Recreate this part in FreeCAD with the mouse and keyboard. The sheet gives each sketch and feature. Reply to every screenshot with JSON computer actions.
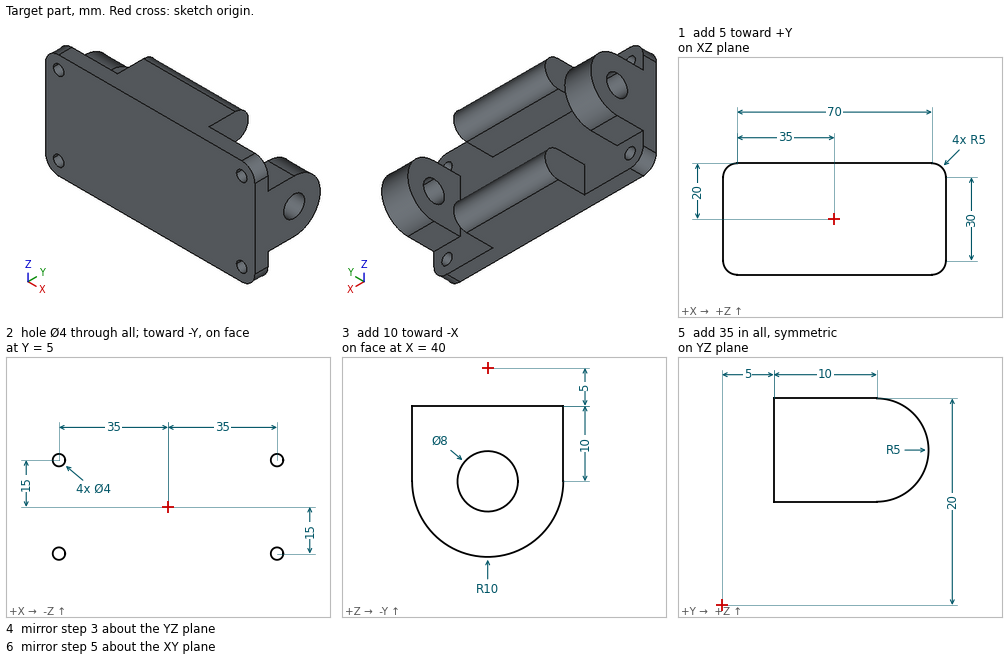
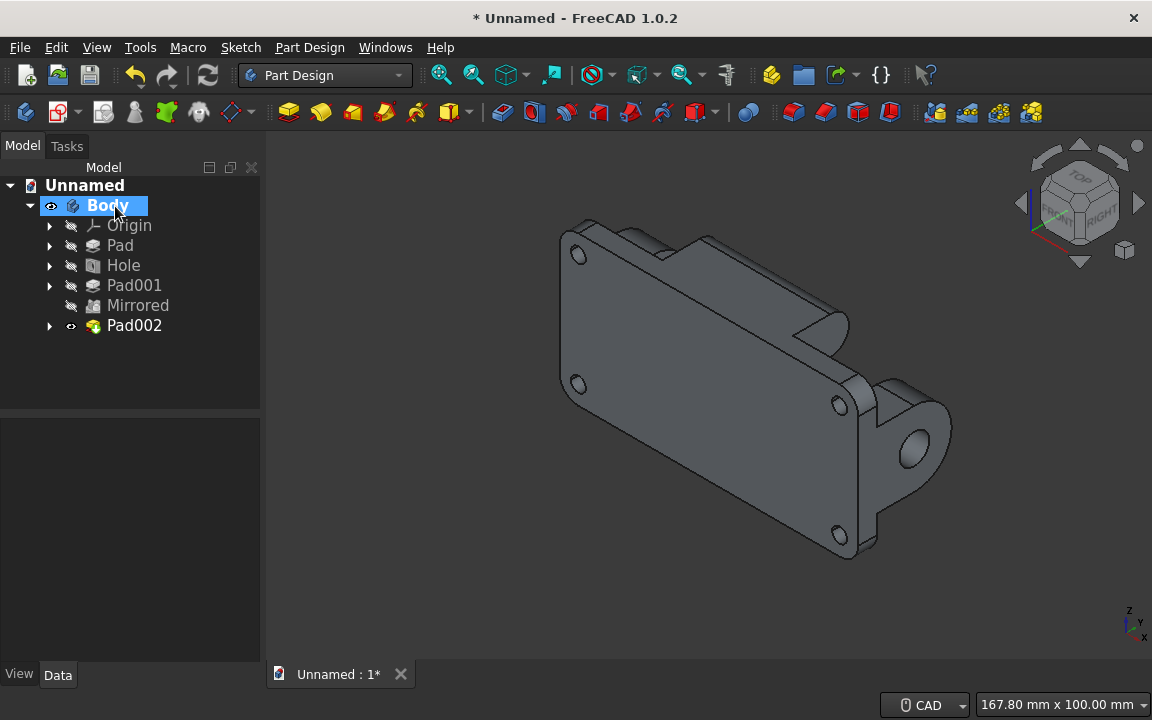
{"action": "left_click", "coordinate": [116, 326]}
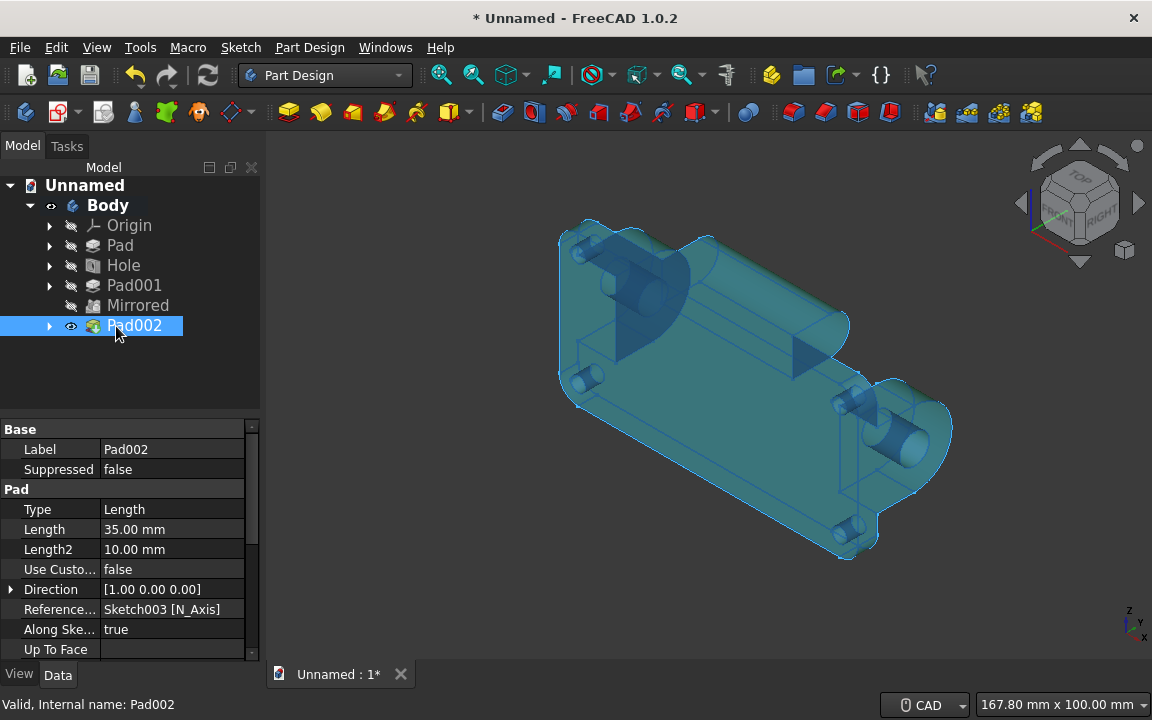
{"action": "left_click", "coordinate": [936, 112]}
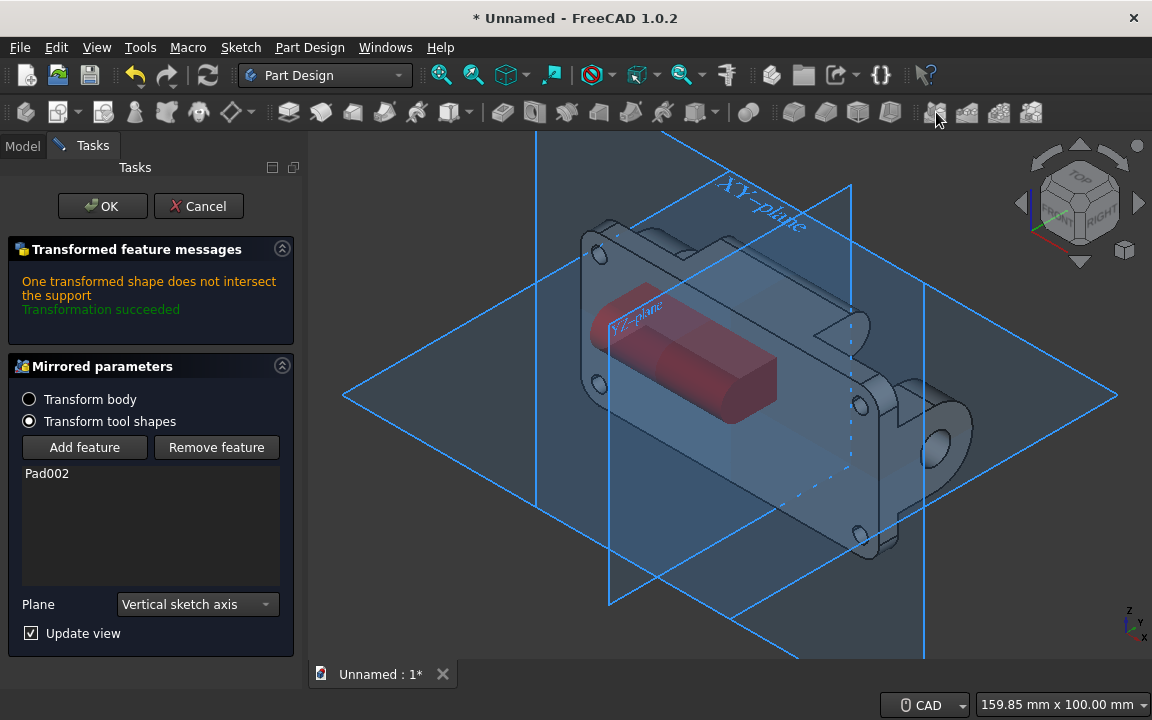
{"action": "left_click", "coordinate": [198, 604]}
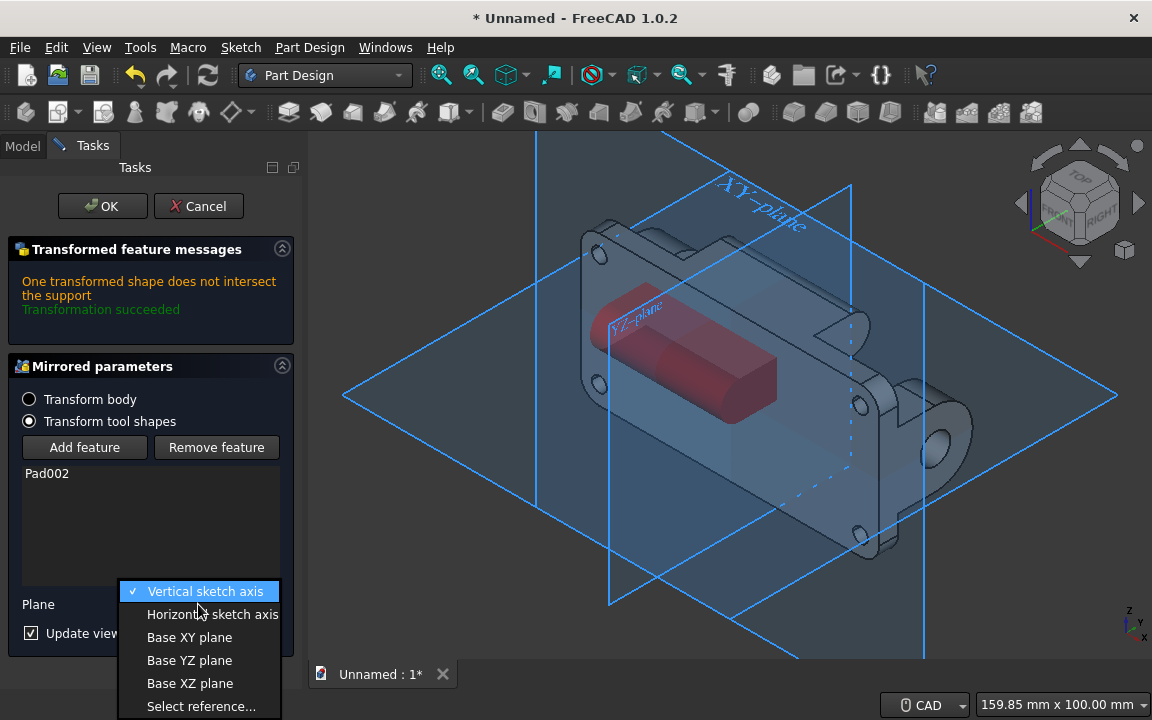
{"action": "left_click", "coordinate": [198, 638]}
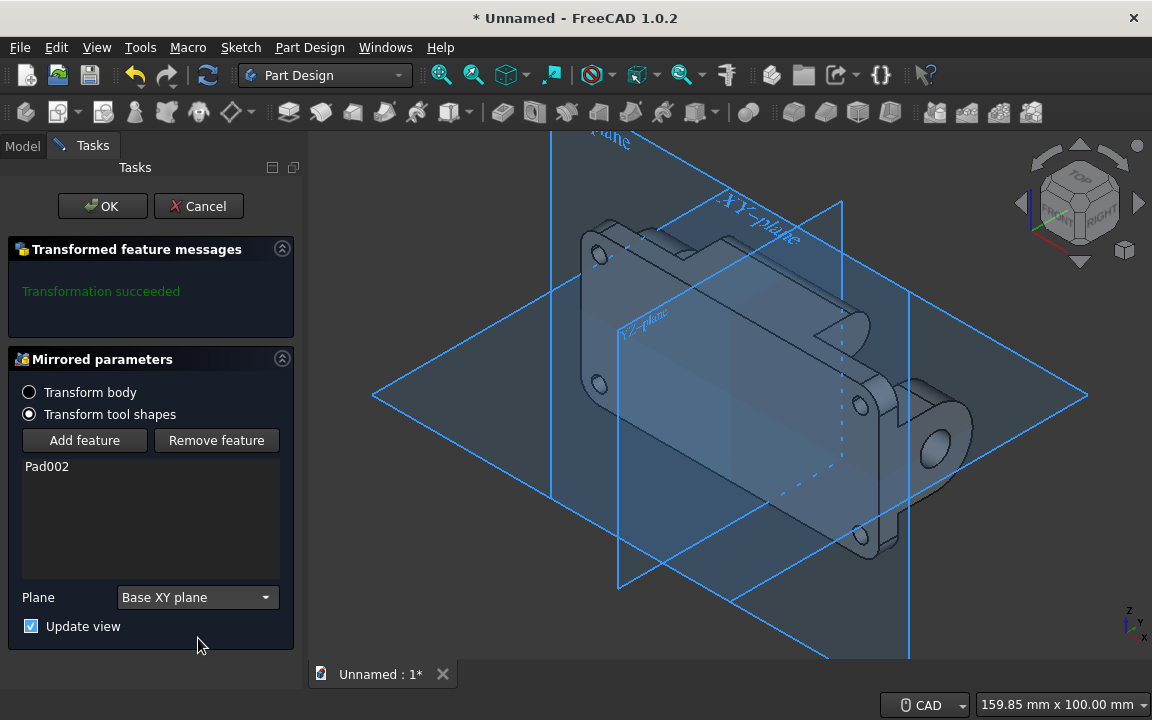
{"action": "left_click", "coordinate": [103, 206]}